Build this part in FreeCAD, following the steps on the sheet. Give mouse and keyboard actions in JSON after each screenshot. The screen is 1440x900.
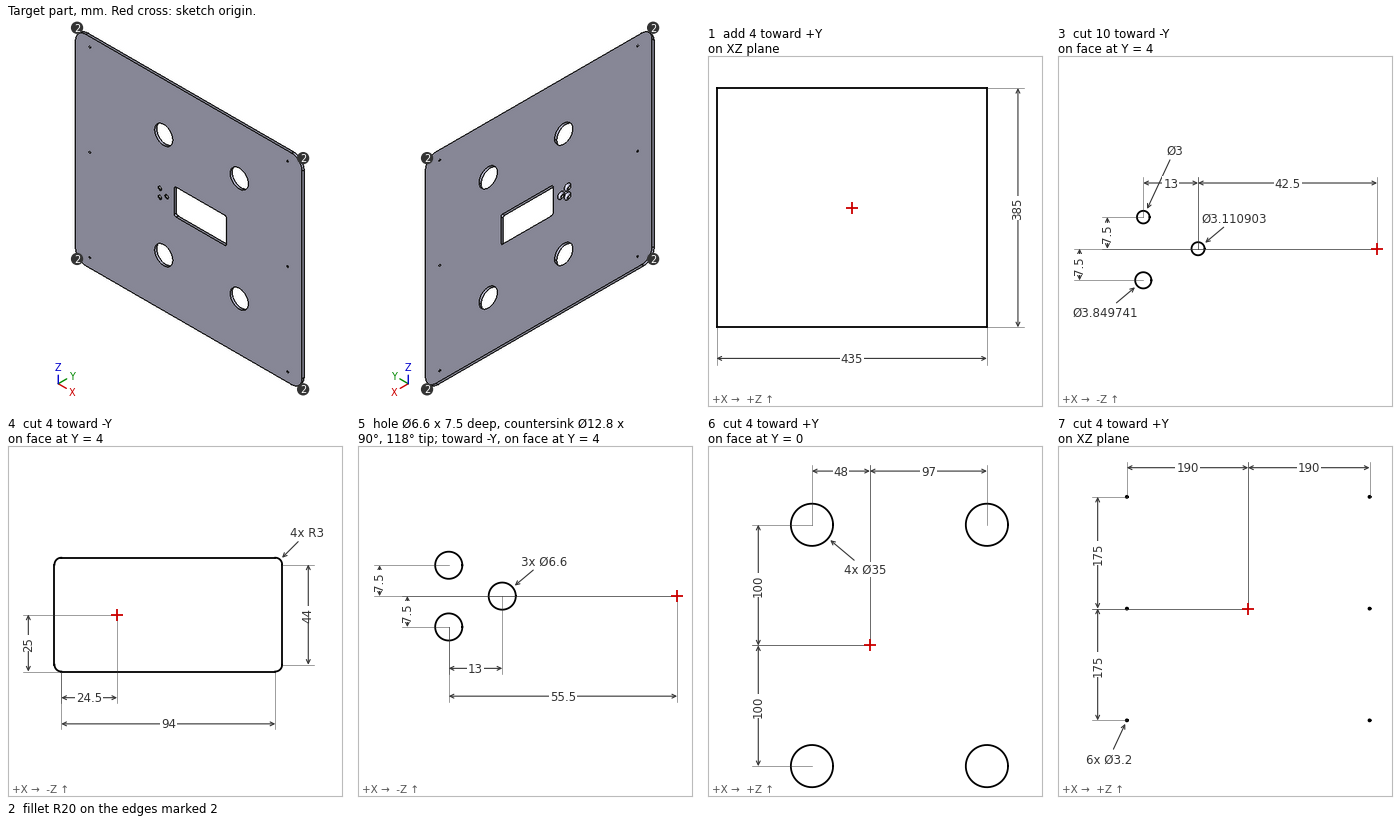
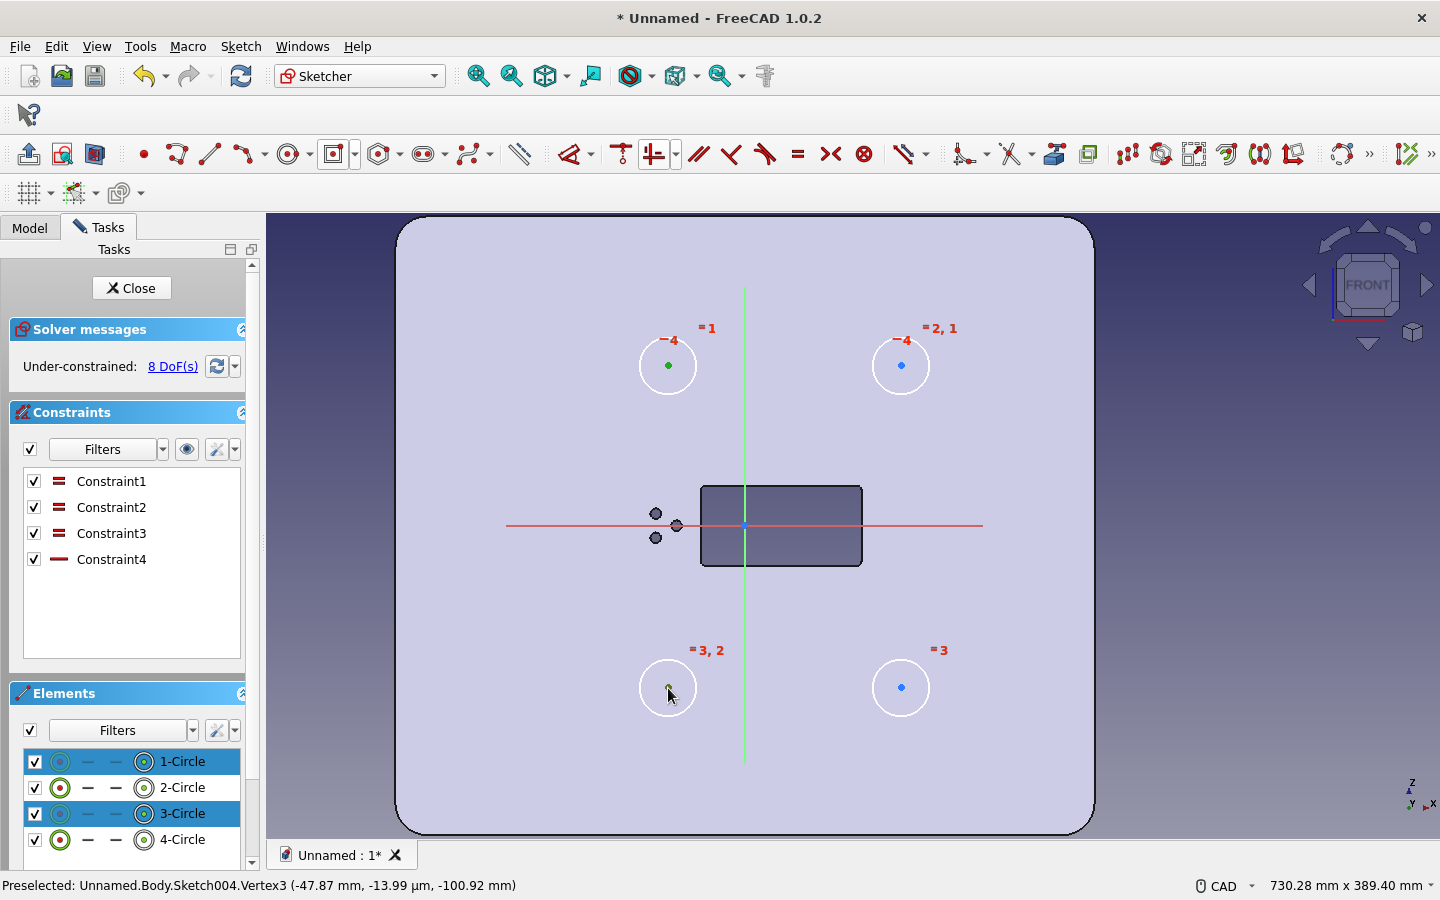
{"action": "left_click", "coordinate": [676, 154]}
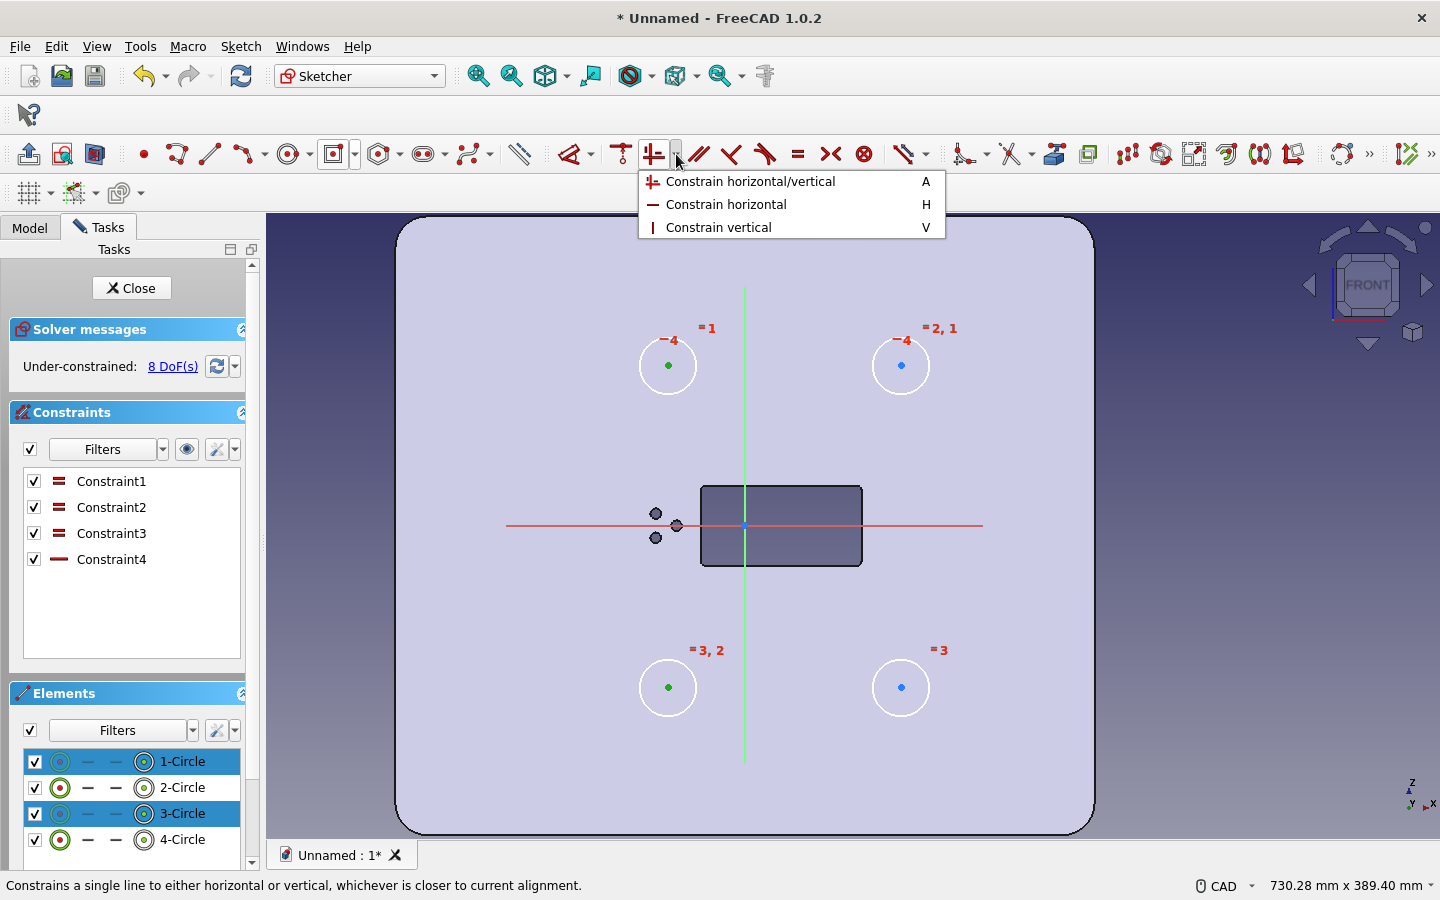
{"action": "left_click", "coordinate": [792, 228]}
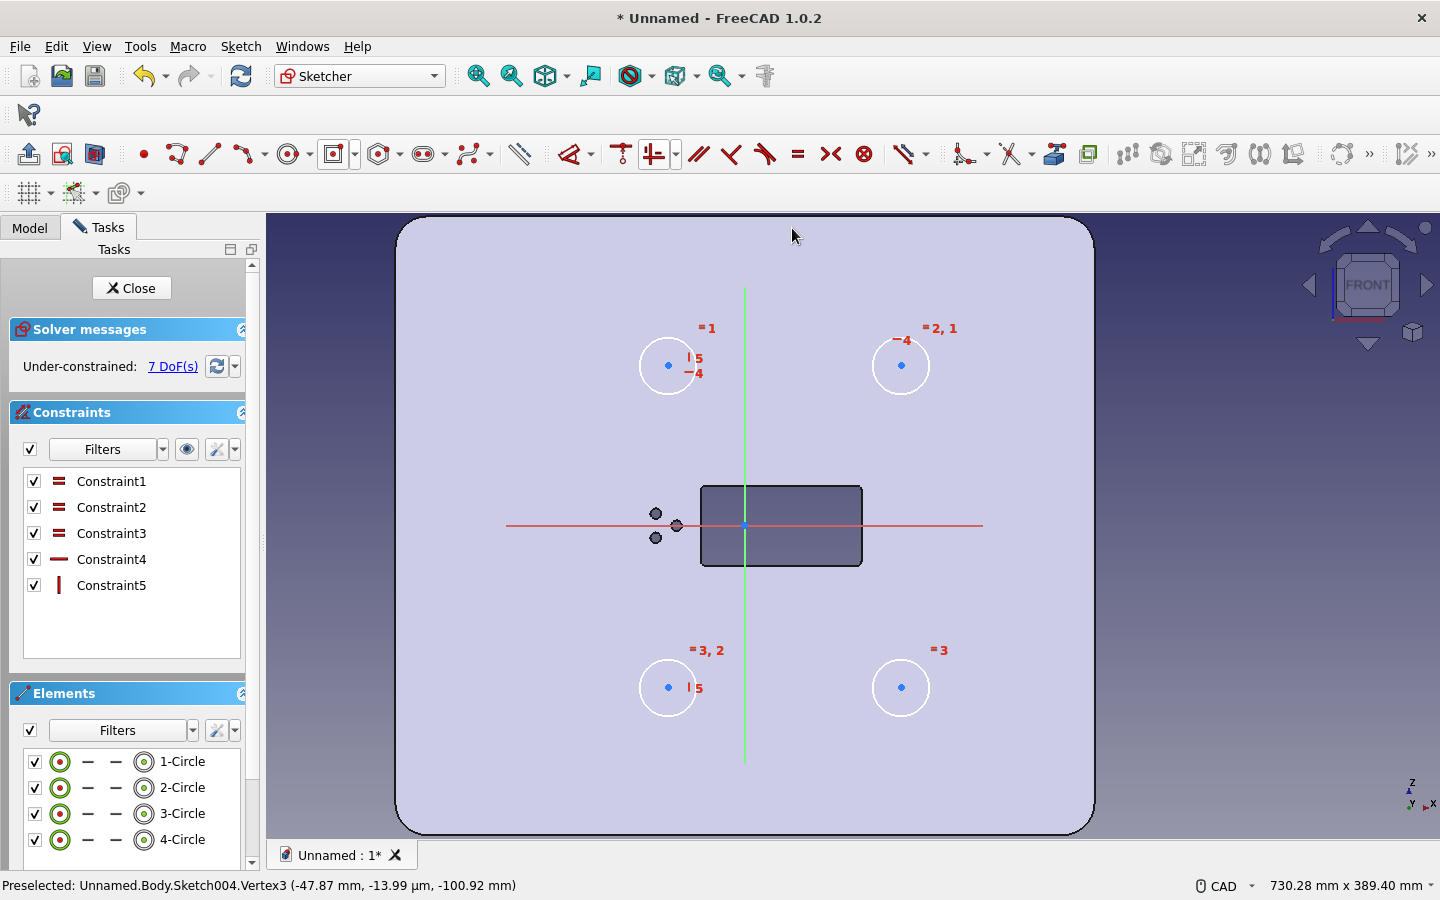
{"action": "left_click", "coordinate": [901, 366]}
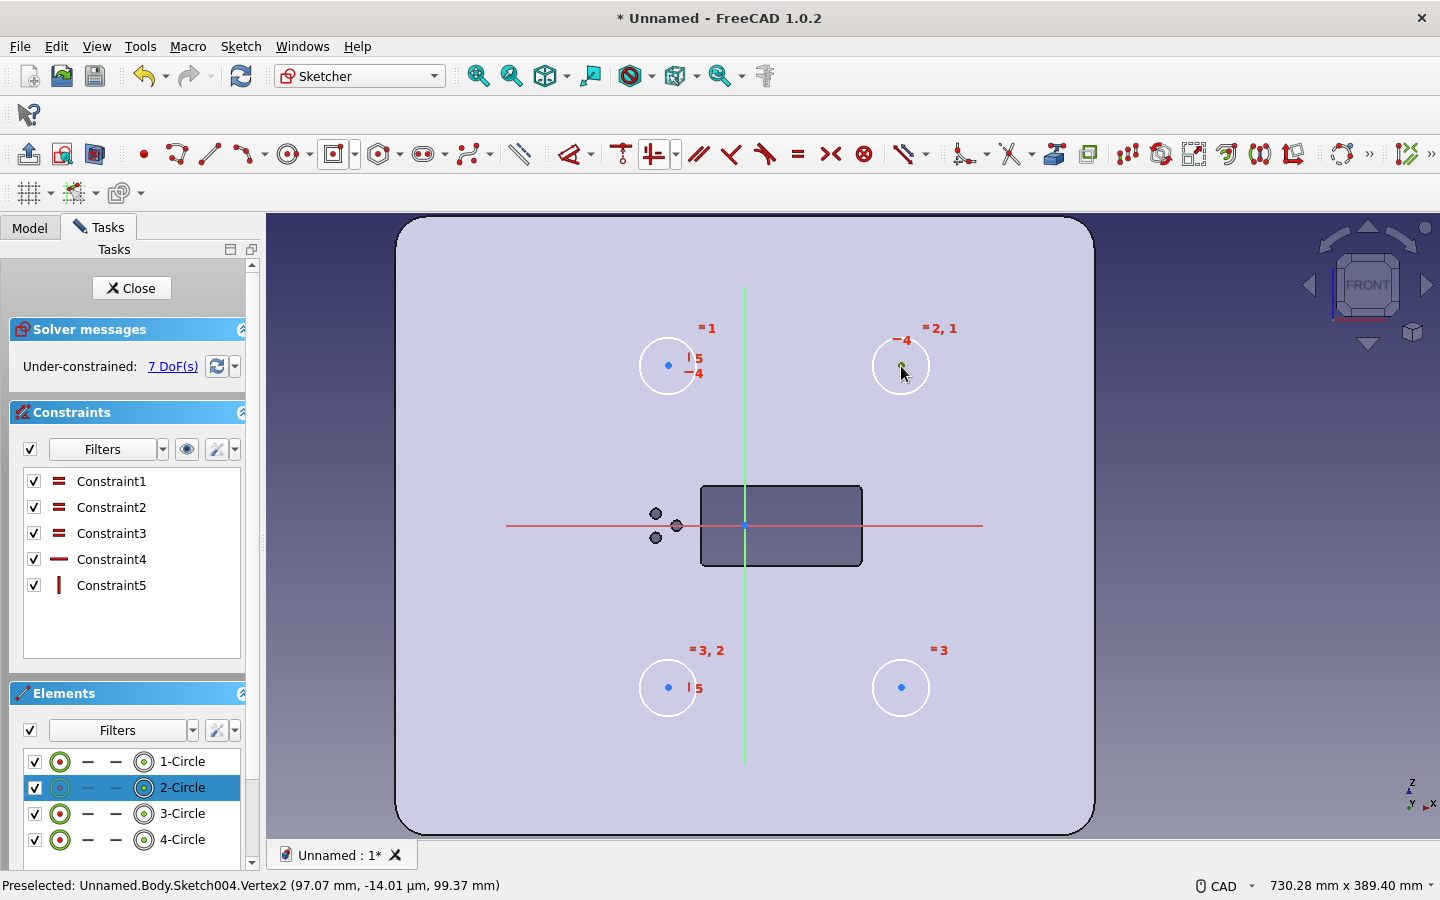
{"action": "left_click", "coordinate": [901, 688]}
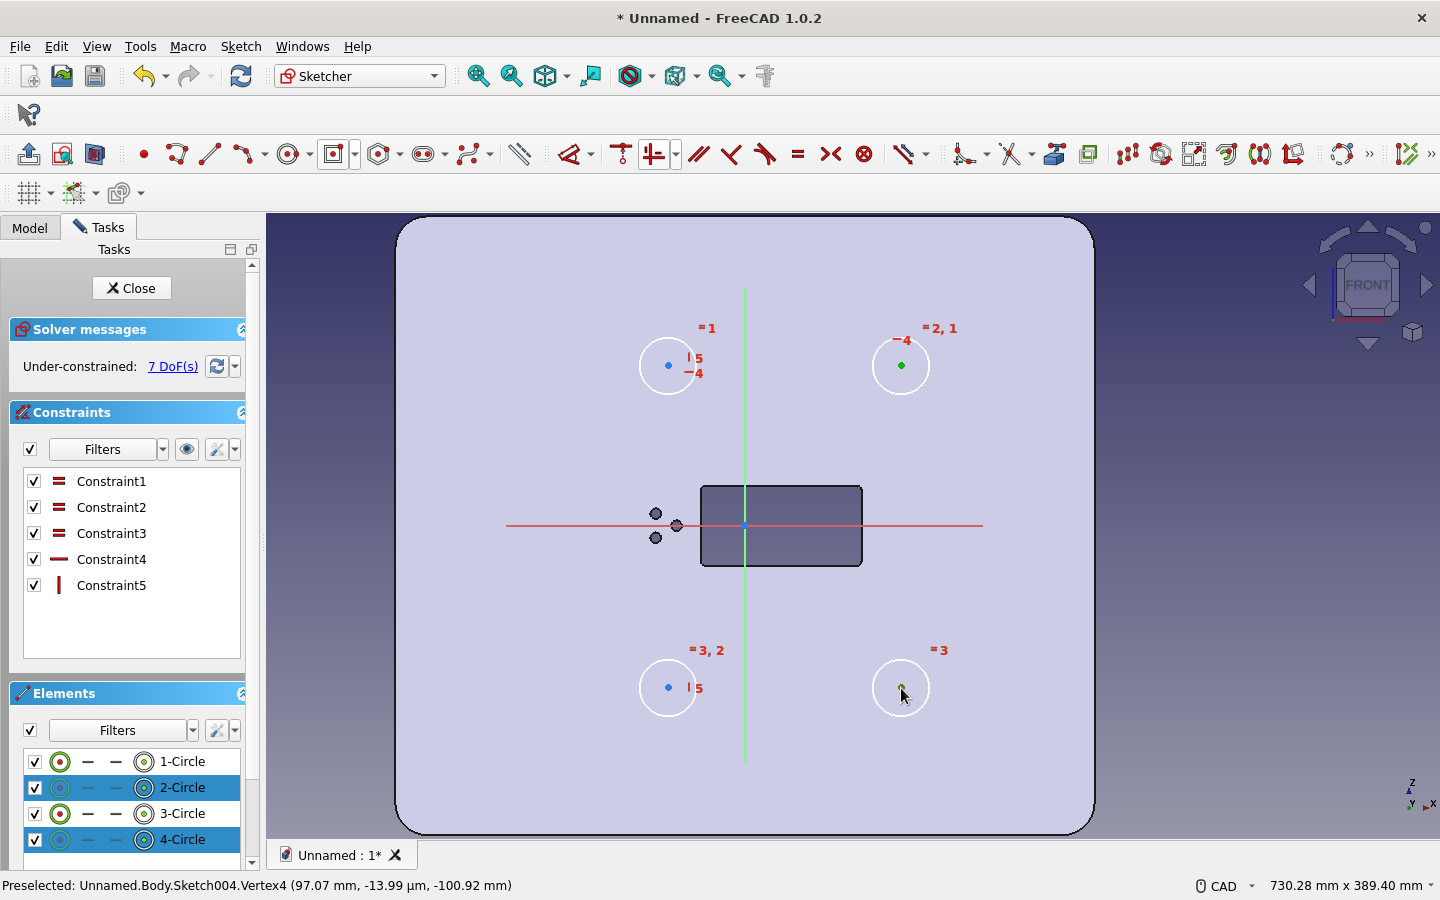
{"action": "left_click", "coordinate": [676, 154]}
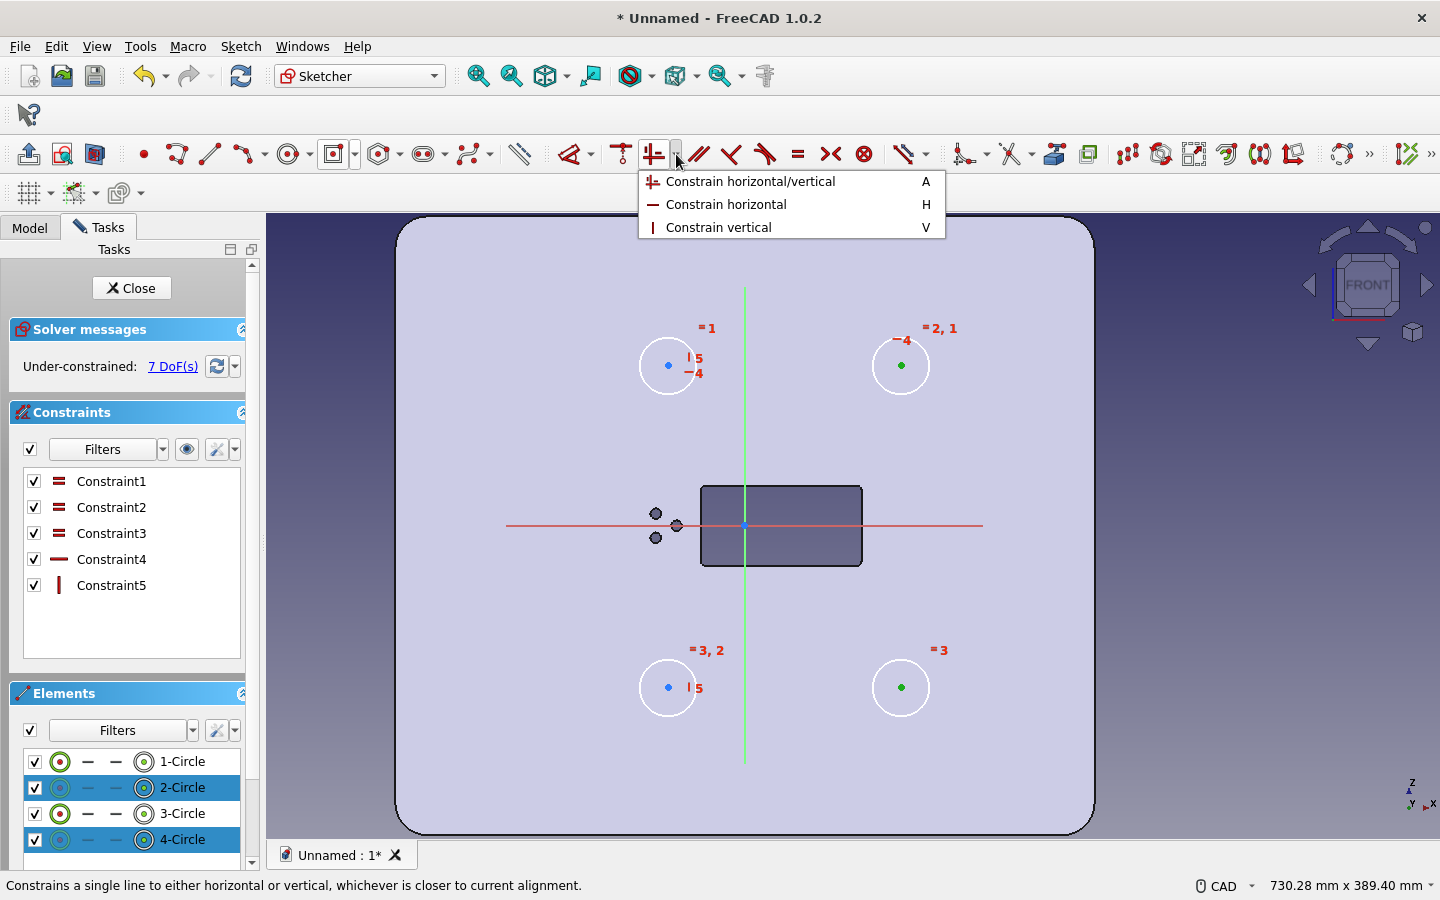
{"action": "left_click", "coordinate": [792, 228]}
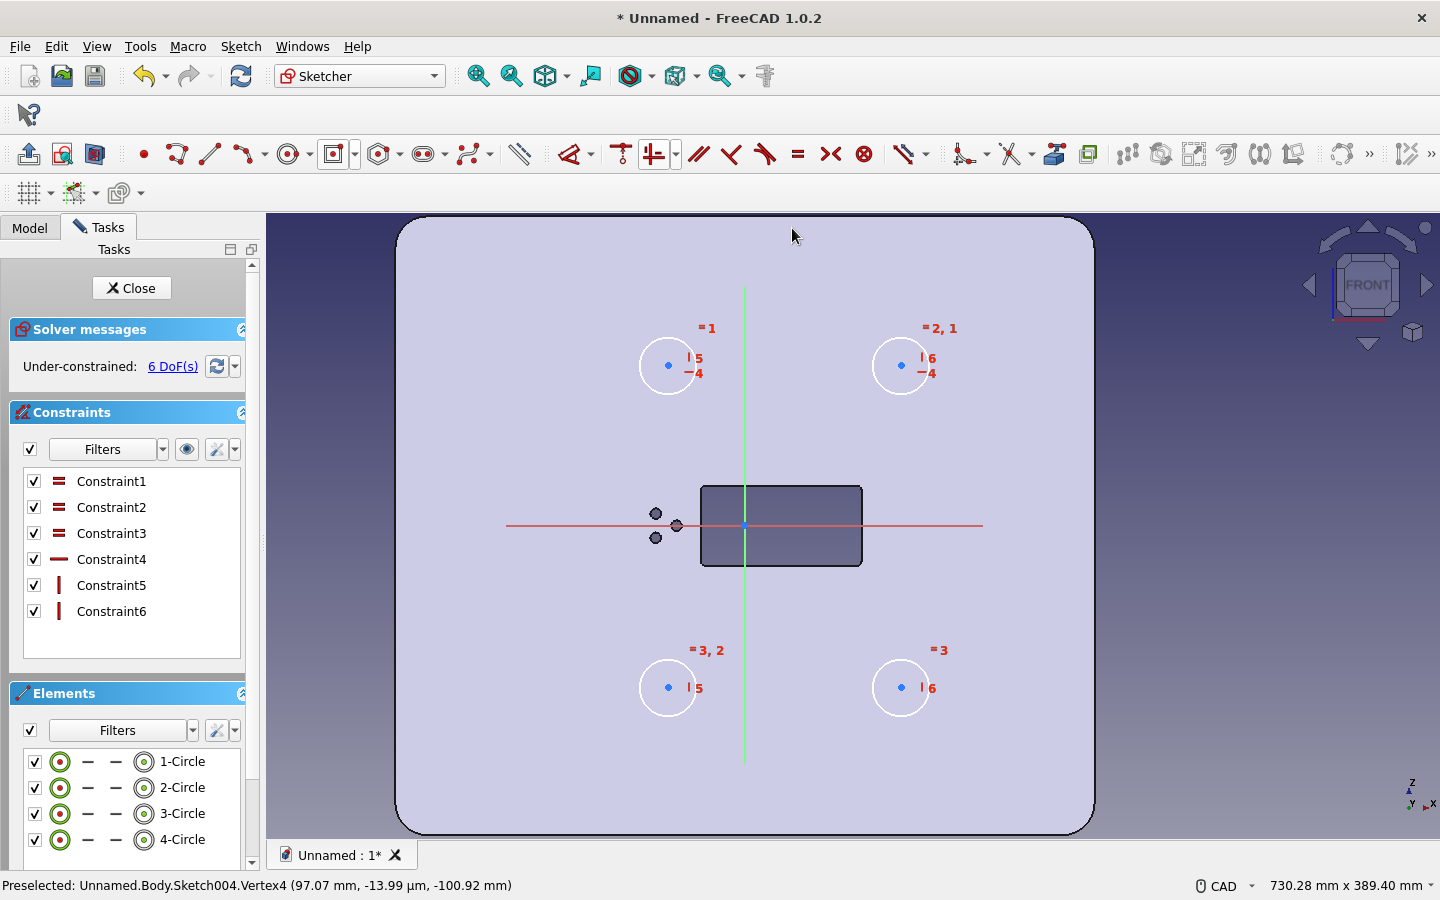
{"action": "left_click", "coordinate": [668, 688]}